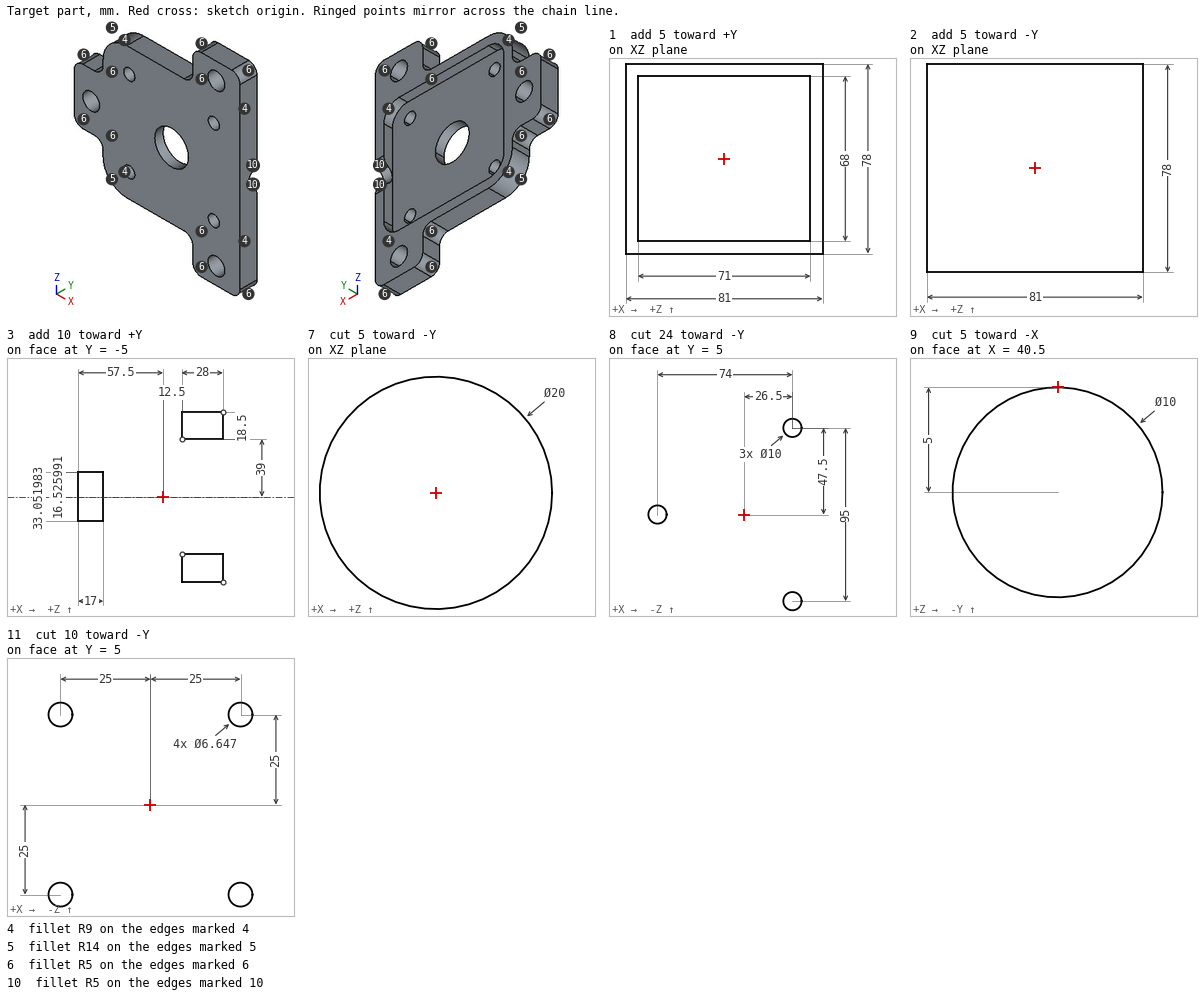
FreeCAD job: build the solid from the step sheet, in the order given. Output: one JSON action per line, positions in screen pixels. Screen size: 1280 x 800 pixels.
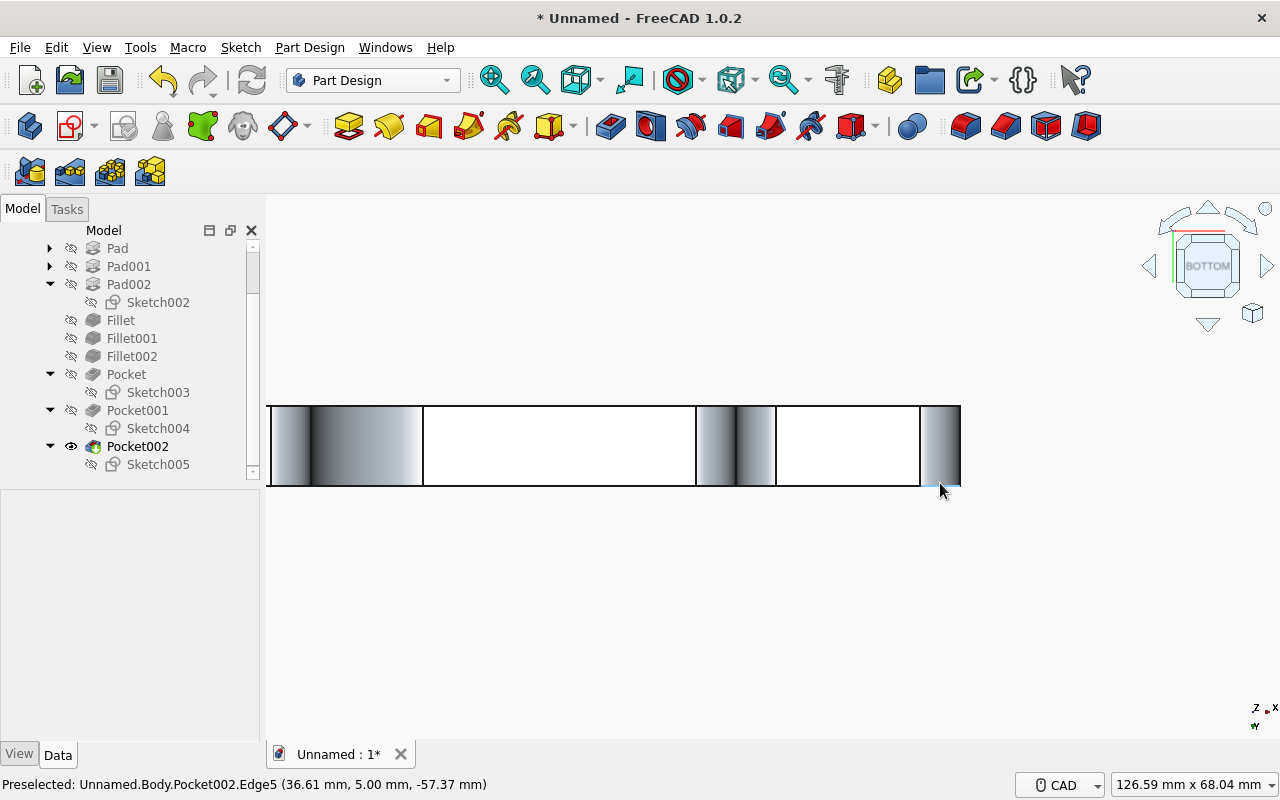
{"action": "key", "text": "v f"}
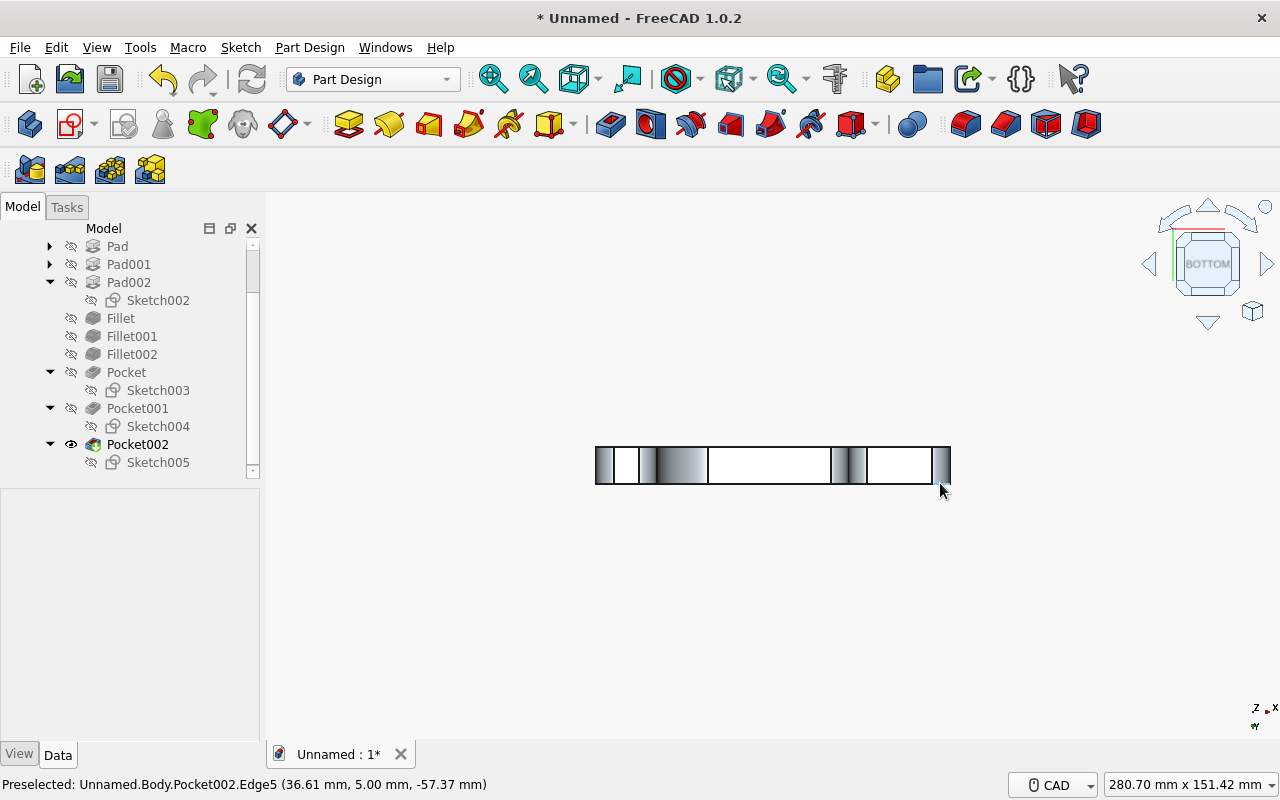
{"action": "key", "text": "4"}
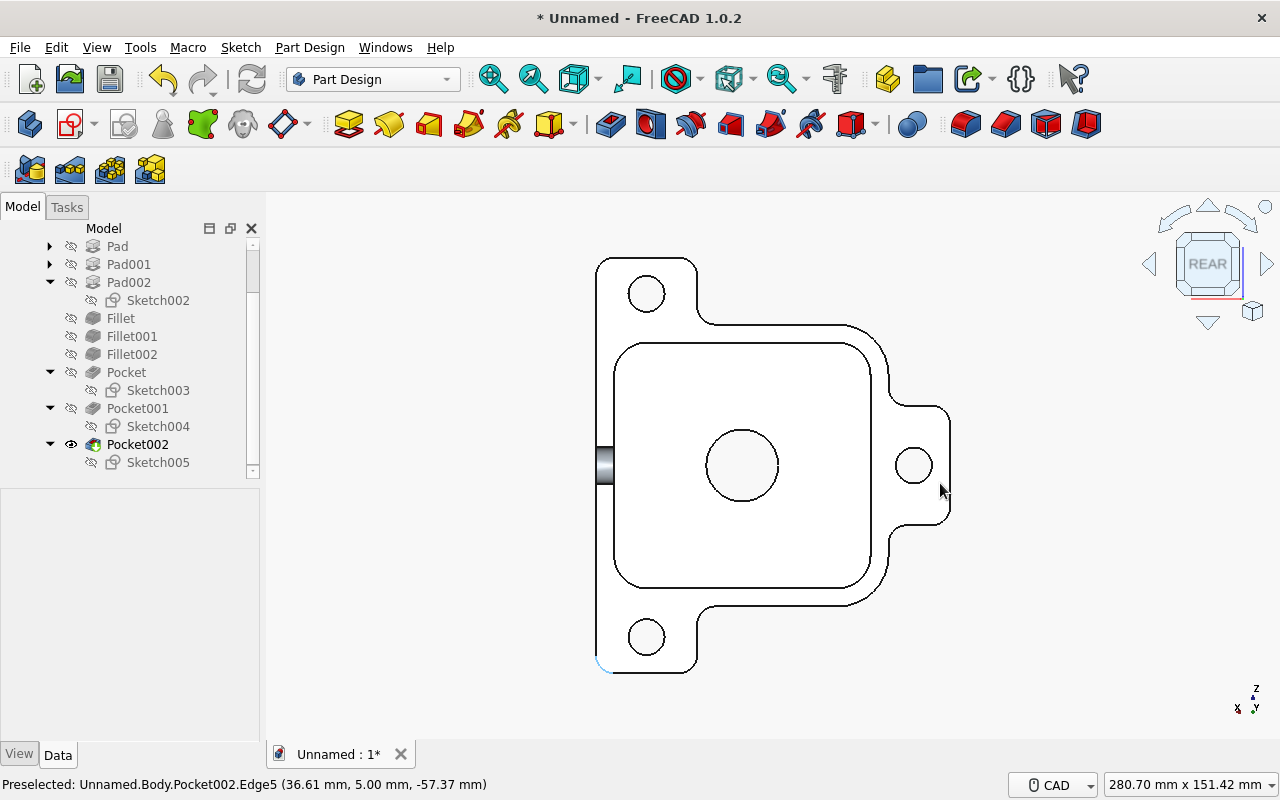
{"action": "left_click", "coordinate": [605, 446]}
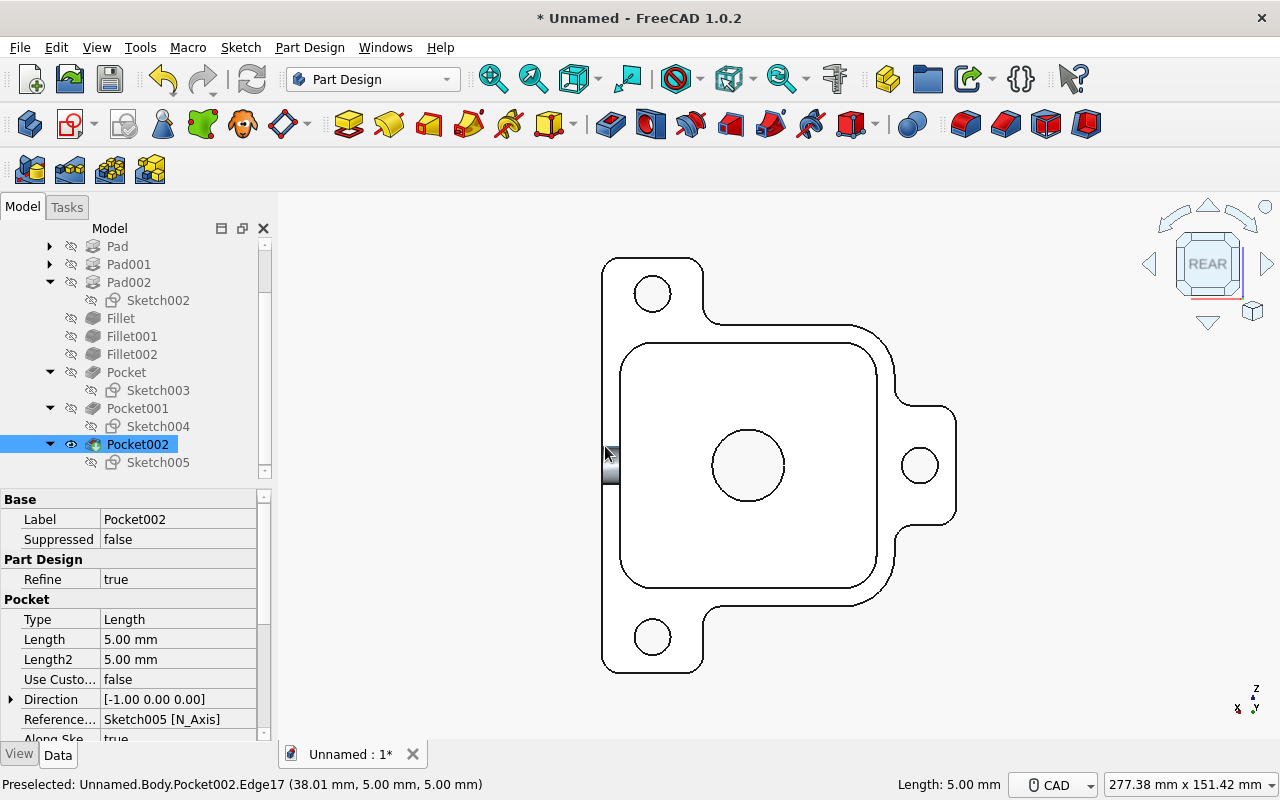
{"action": "scroll", "coordinate": [611, 483], "scroll_direction": "up", "scroll_amount": 4}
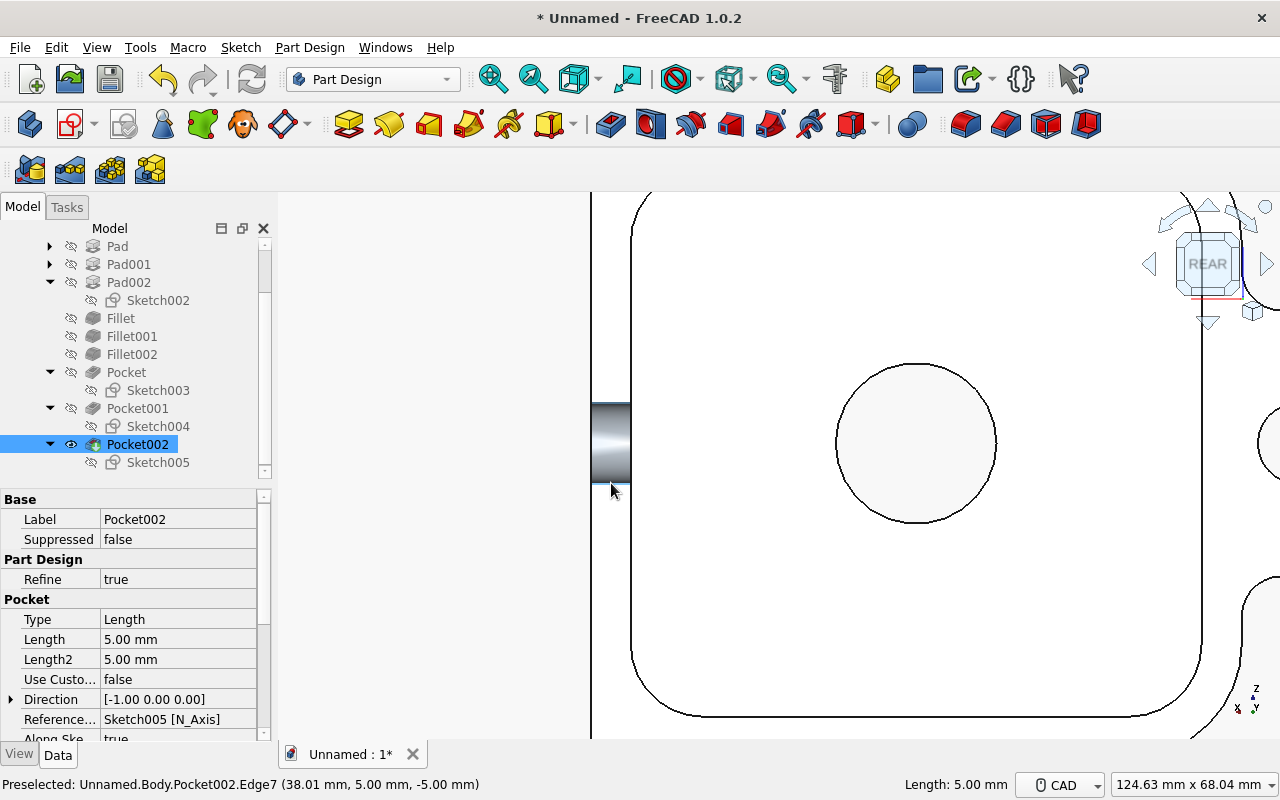
{"action": "left_click", "coordinate": [494, 80]}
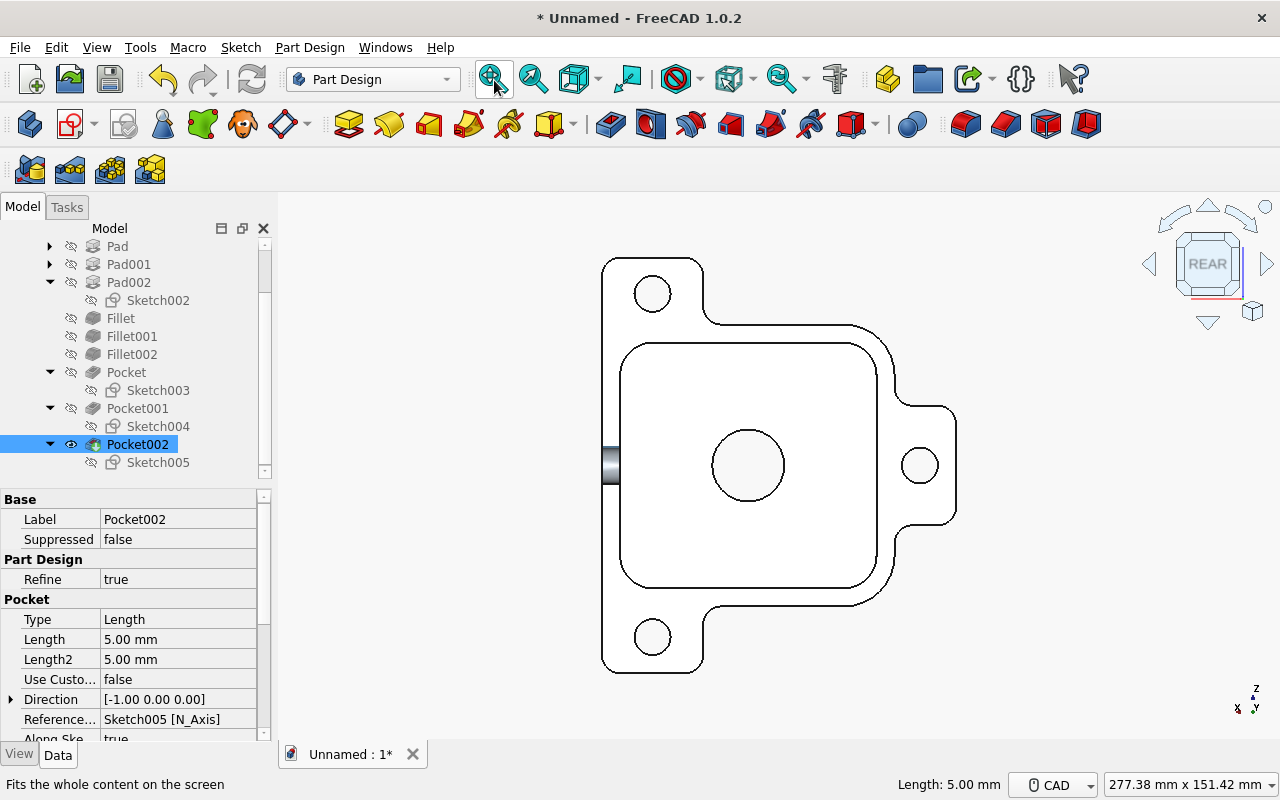
{"action": "key", "text": "6"}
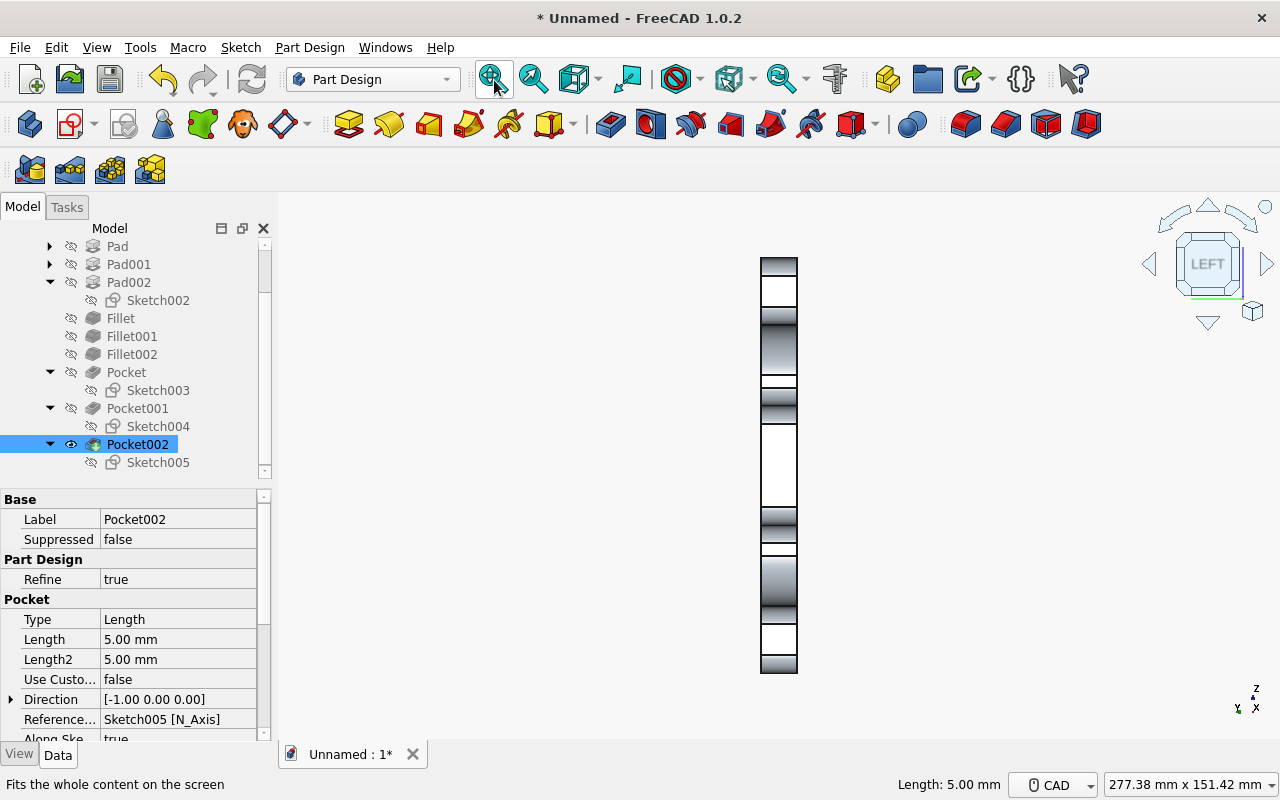
{"action": "scroll", "coordinate": [761, 483], "scroll_direction": "up", "scroll_amount": 4}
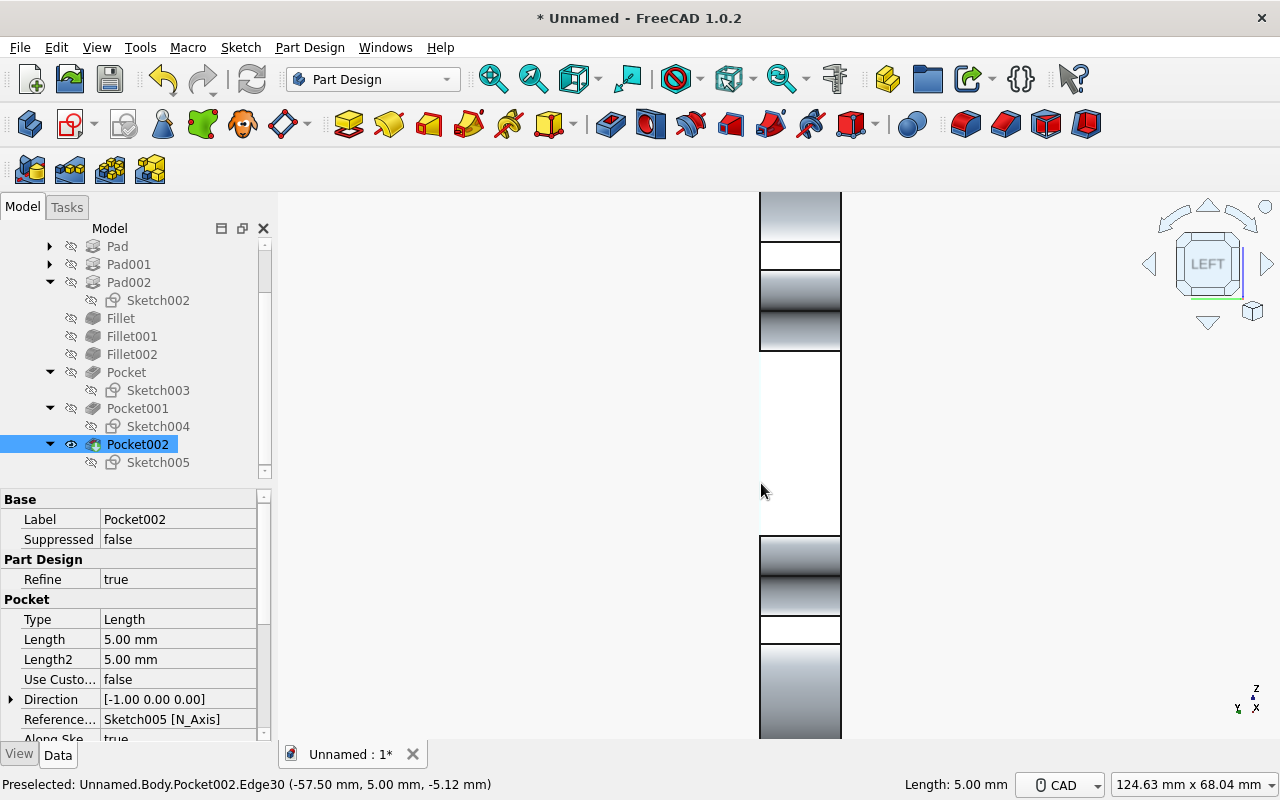
{"action": "left_click", "coordinate": [494, 80]}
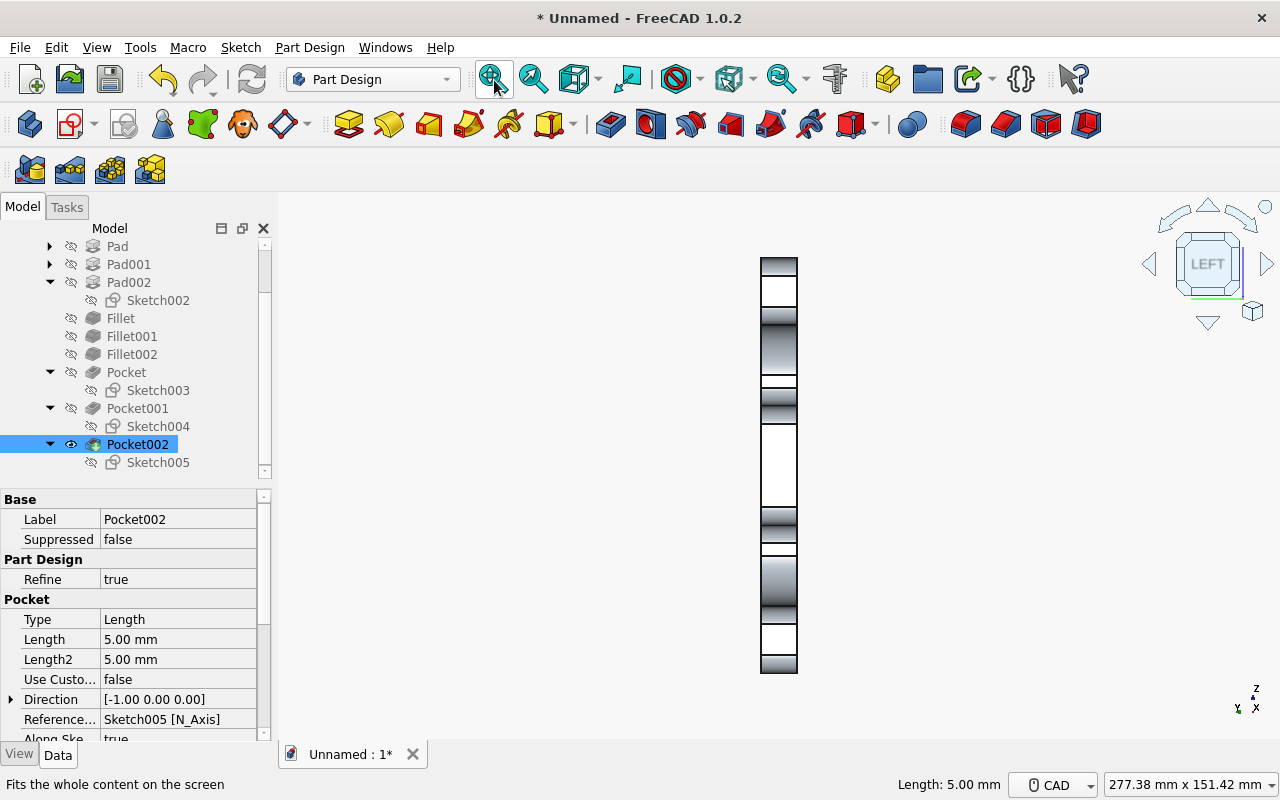
{"action": "key", "text": "v 3"}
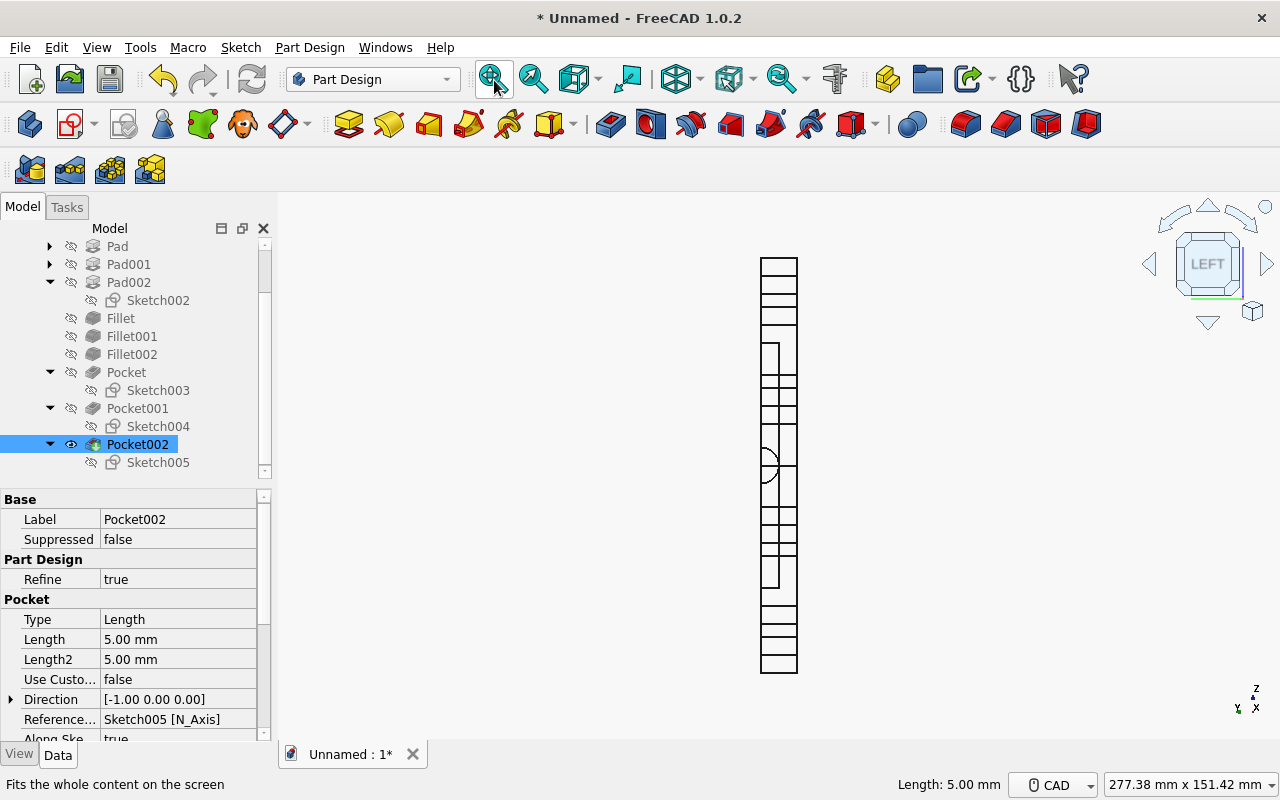
{"action": "key", "text": "0"}